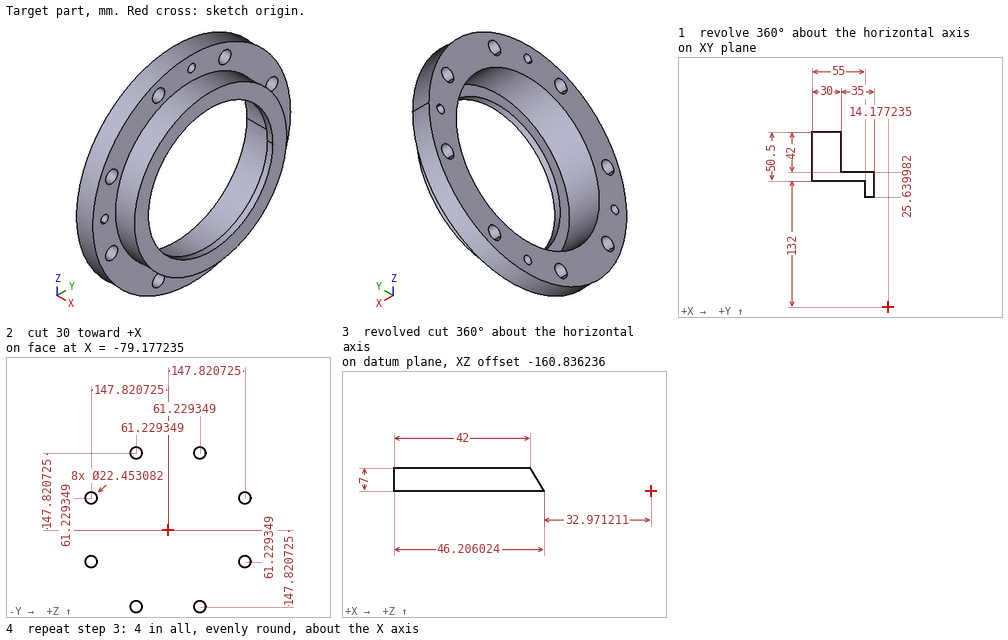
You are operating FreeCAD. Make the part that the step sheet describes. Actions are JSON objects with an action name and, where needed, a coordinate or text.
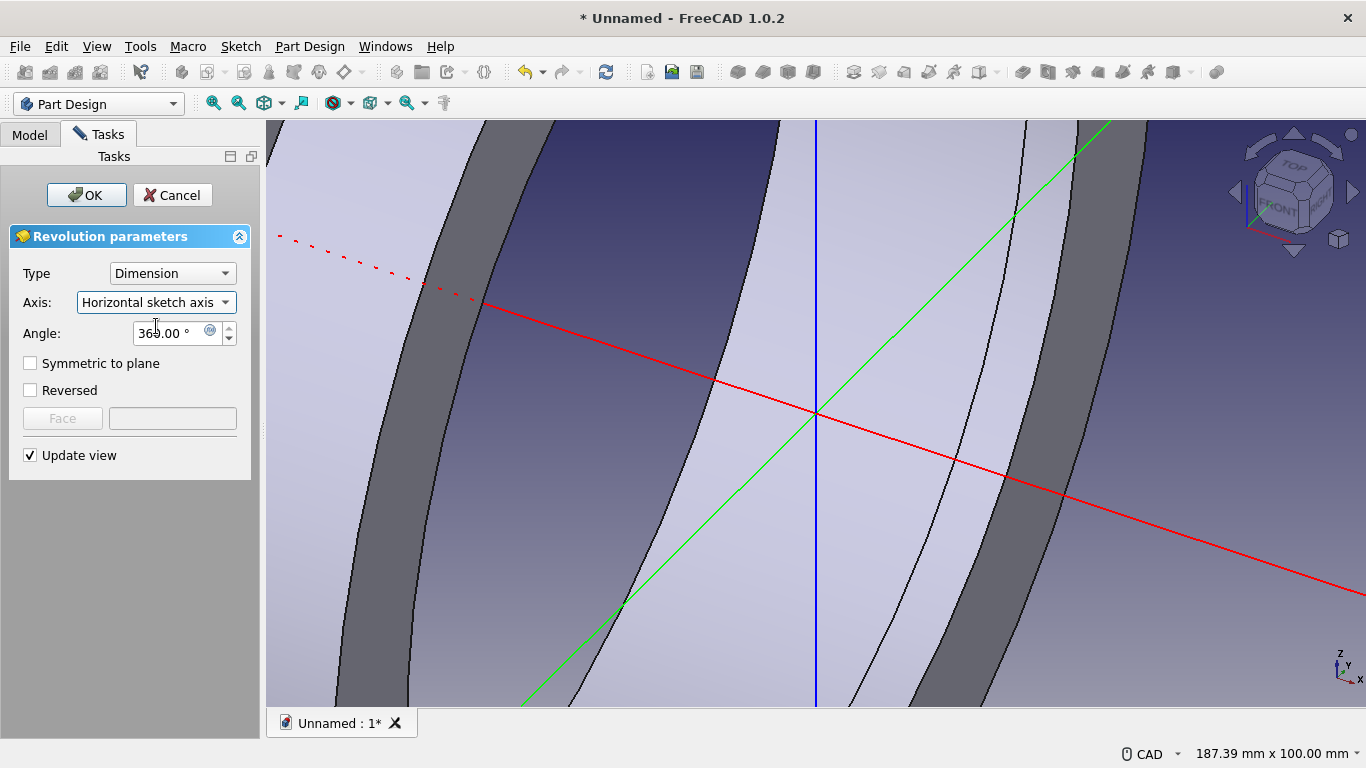
{"action": "left_click", "coordinate": [87, 195]}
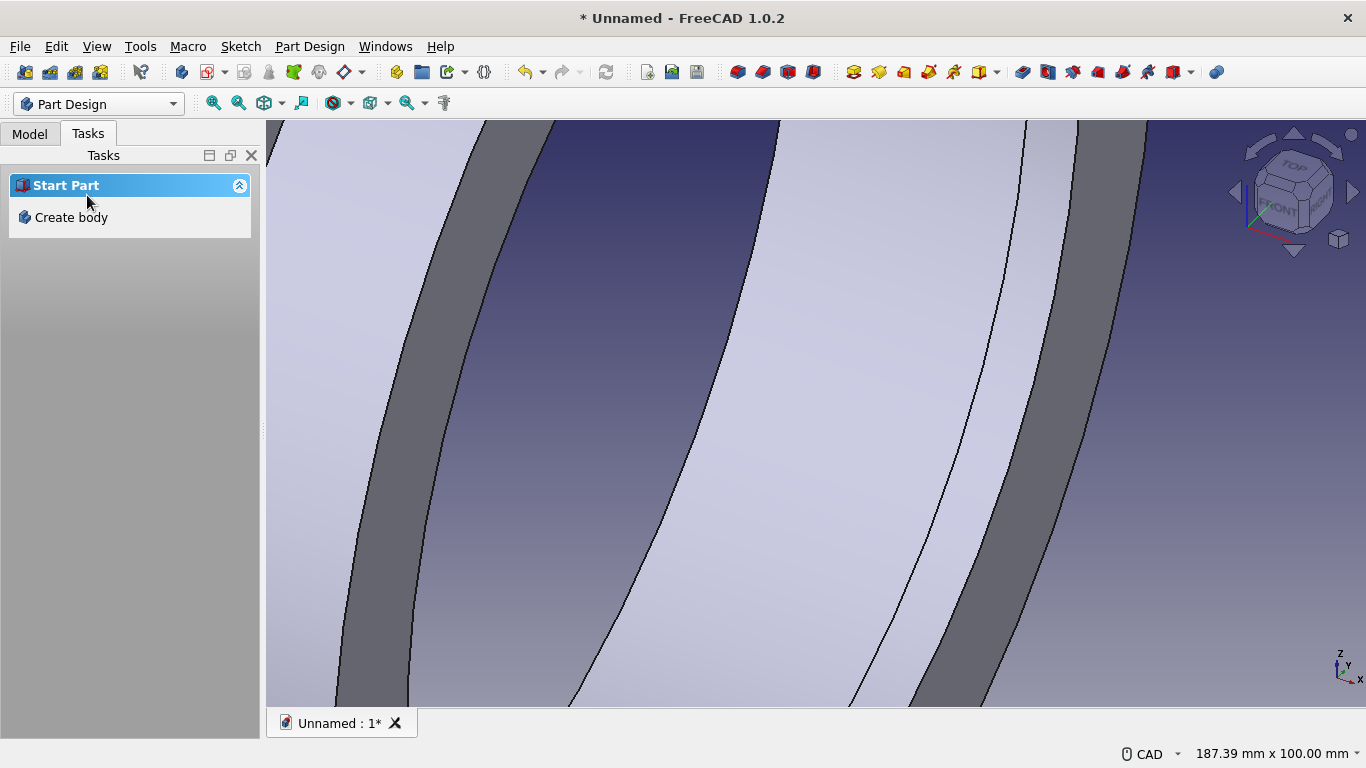
{"action": "left_click", "coordinate": [214, 104]}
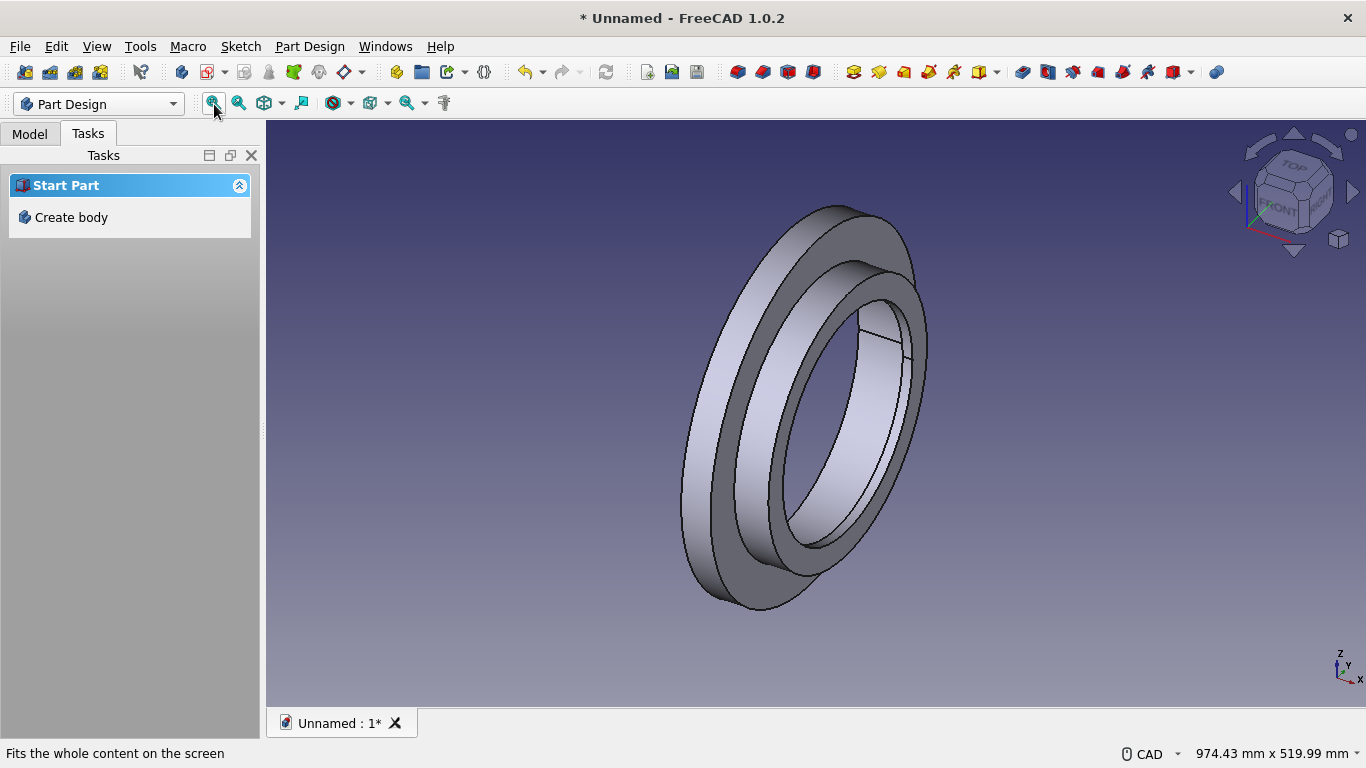
{"action": "key", "text": "6"}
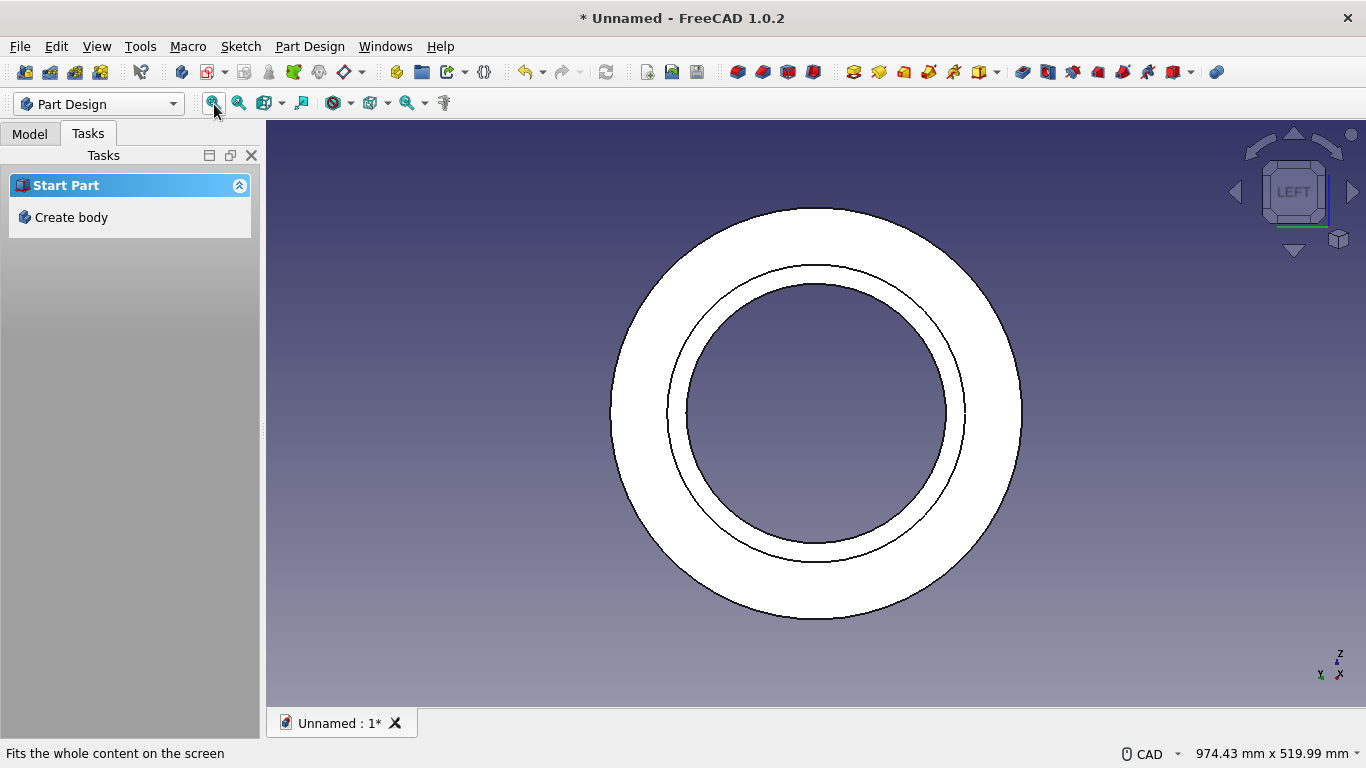
{"action": "left_click", "coordinate": [640, 412]}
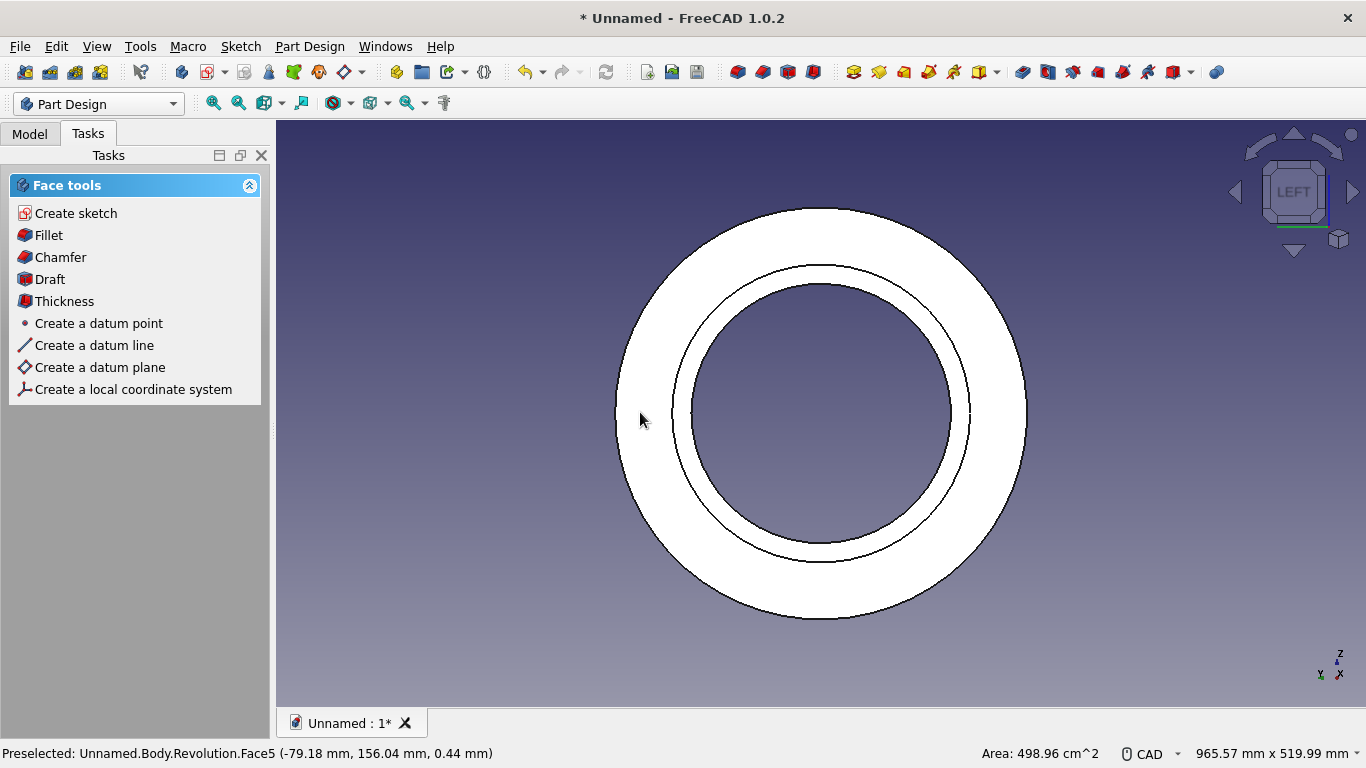
{"action": "left_click", "coordinate": [206, 72]}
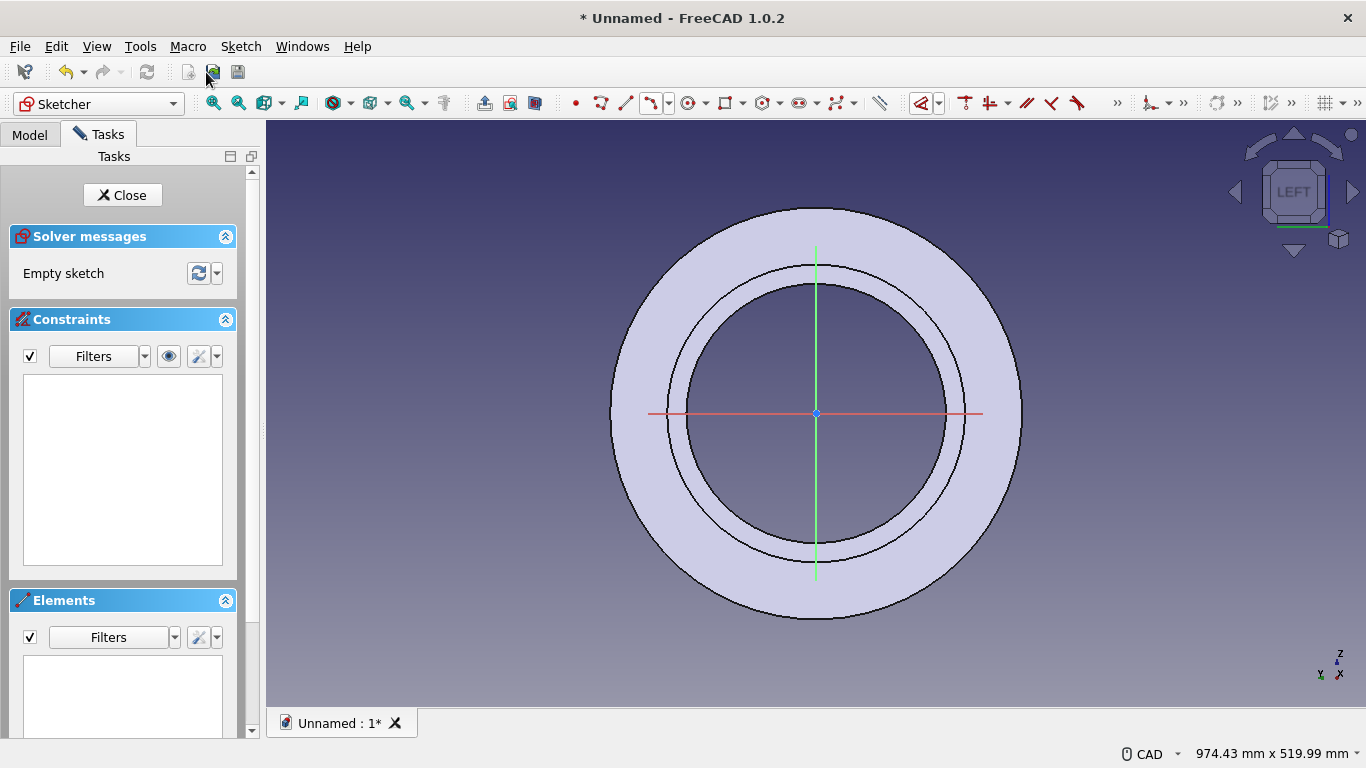
{"action": "left_click", "coordinate": [688, 104]}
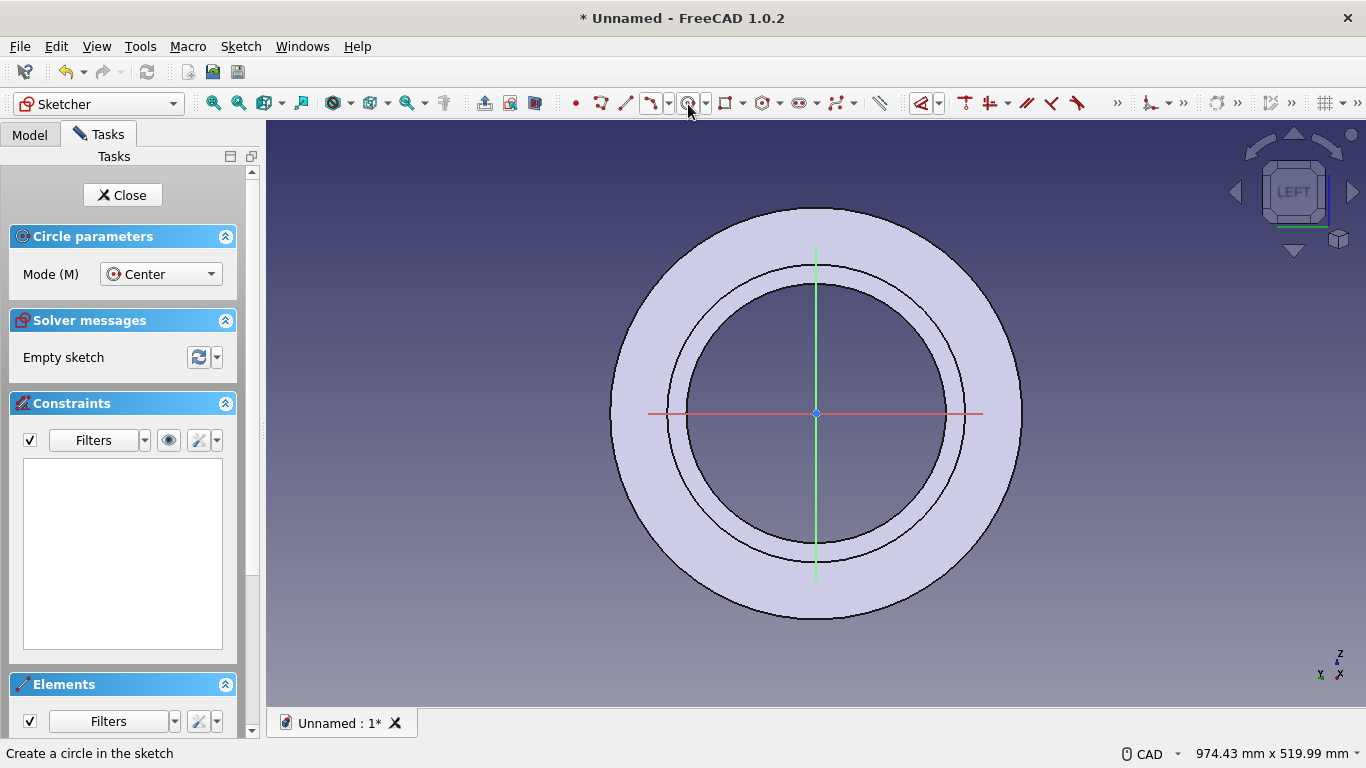
{"action": "scroll", "coordinate": [649, 344], "scroll_direction": "up", "scroll_amount": 3}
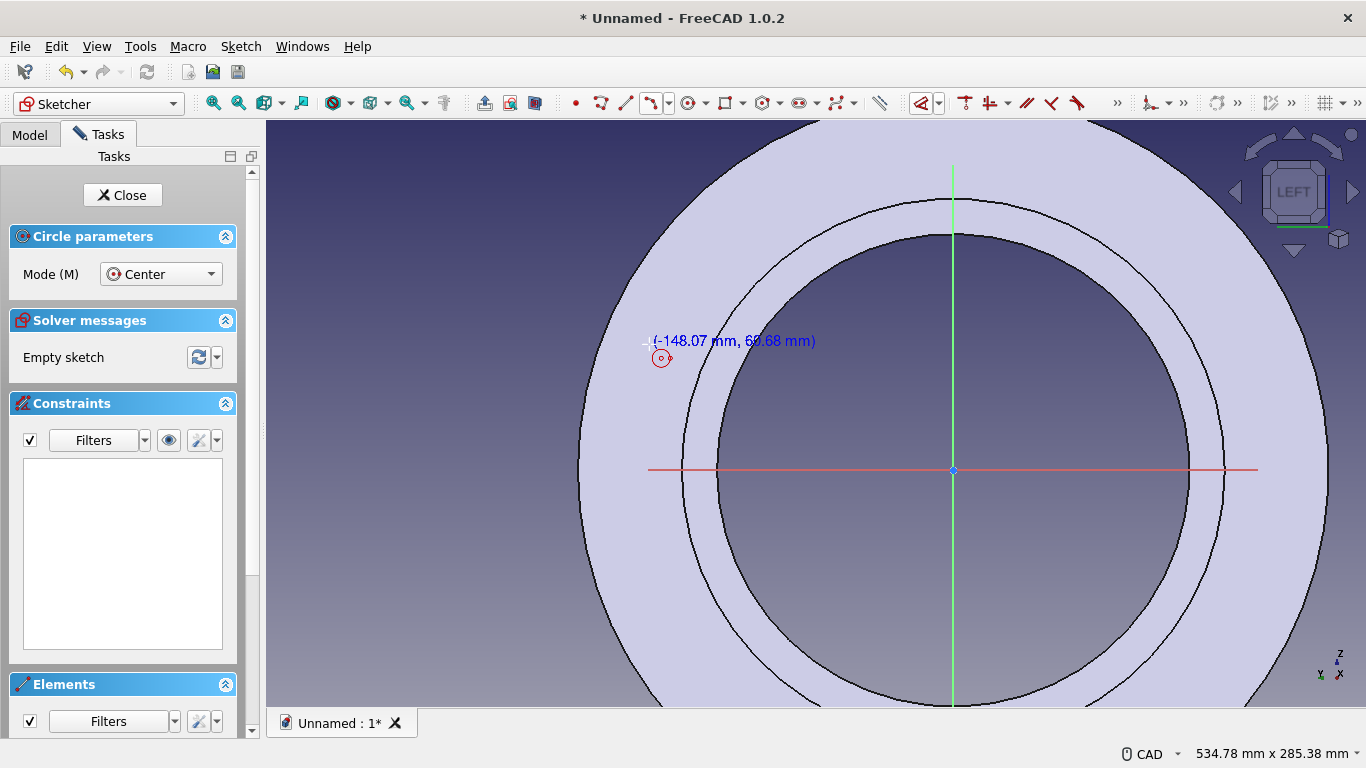
{"action": "left_click", "coordinate": [649, 344]}
{"action": "mouse_move", "coordinate": [666, 328]}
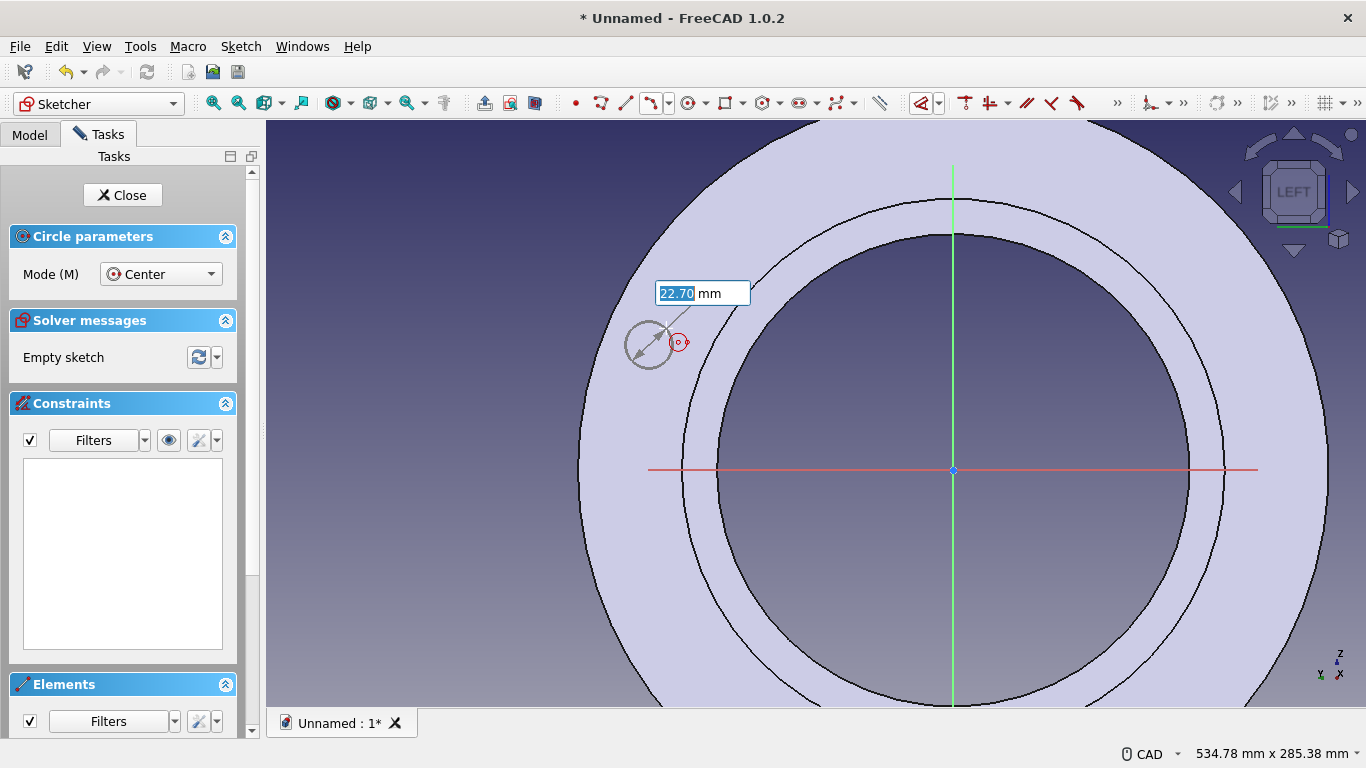
{"action": "type", "text": "22.453082"}
{"action": "key", "text": "Return"}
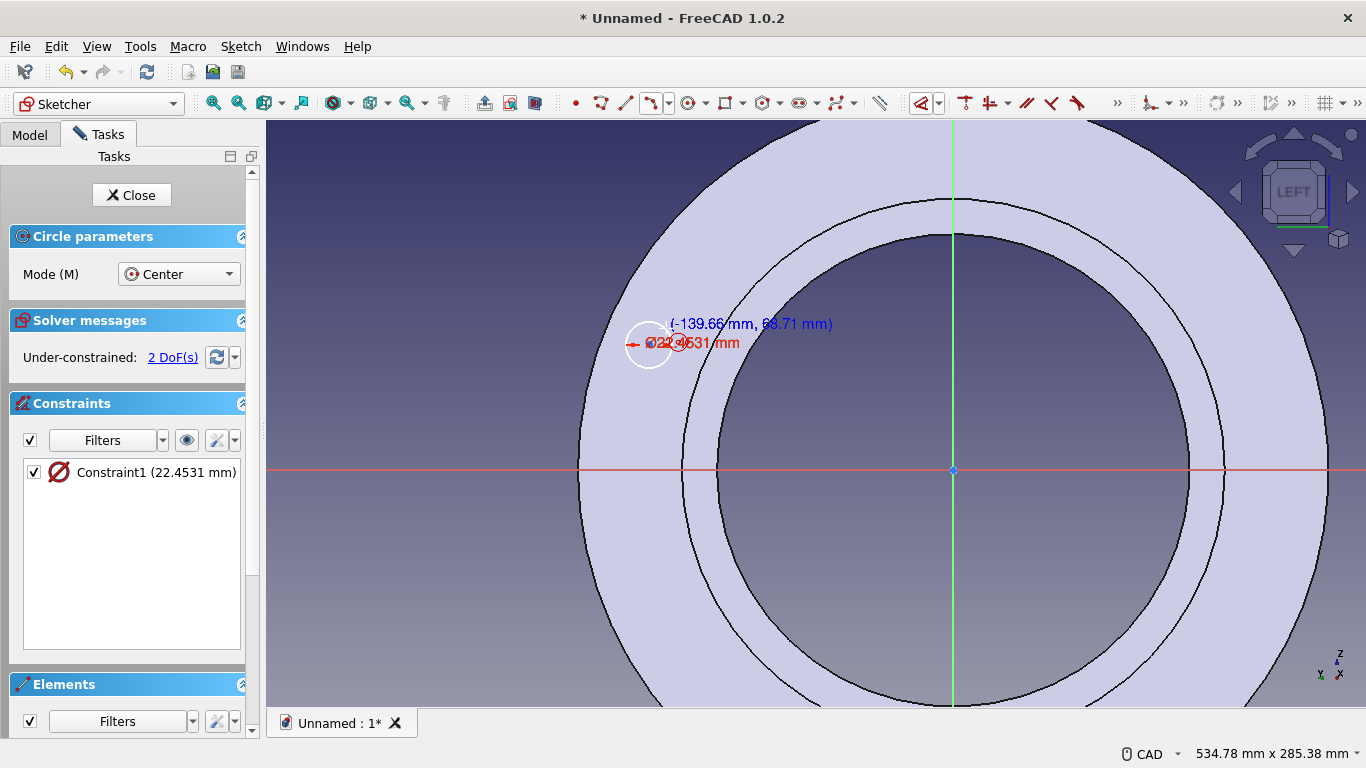
{"action": "left_click", "coordinate": [827, 166]}
{"action": "mouse_move", "coordinate": [844, 150]}